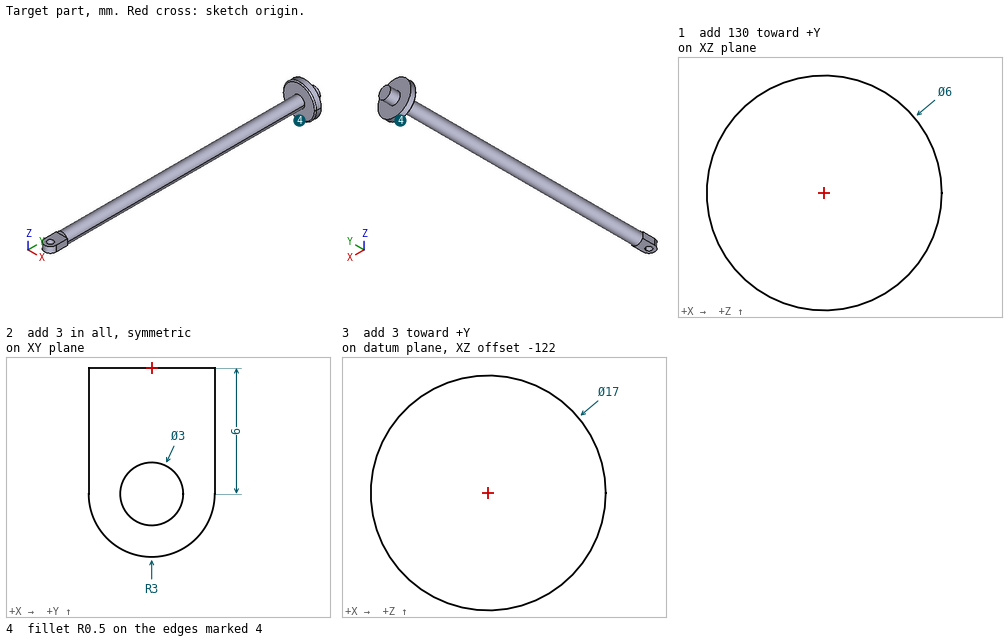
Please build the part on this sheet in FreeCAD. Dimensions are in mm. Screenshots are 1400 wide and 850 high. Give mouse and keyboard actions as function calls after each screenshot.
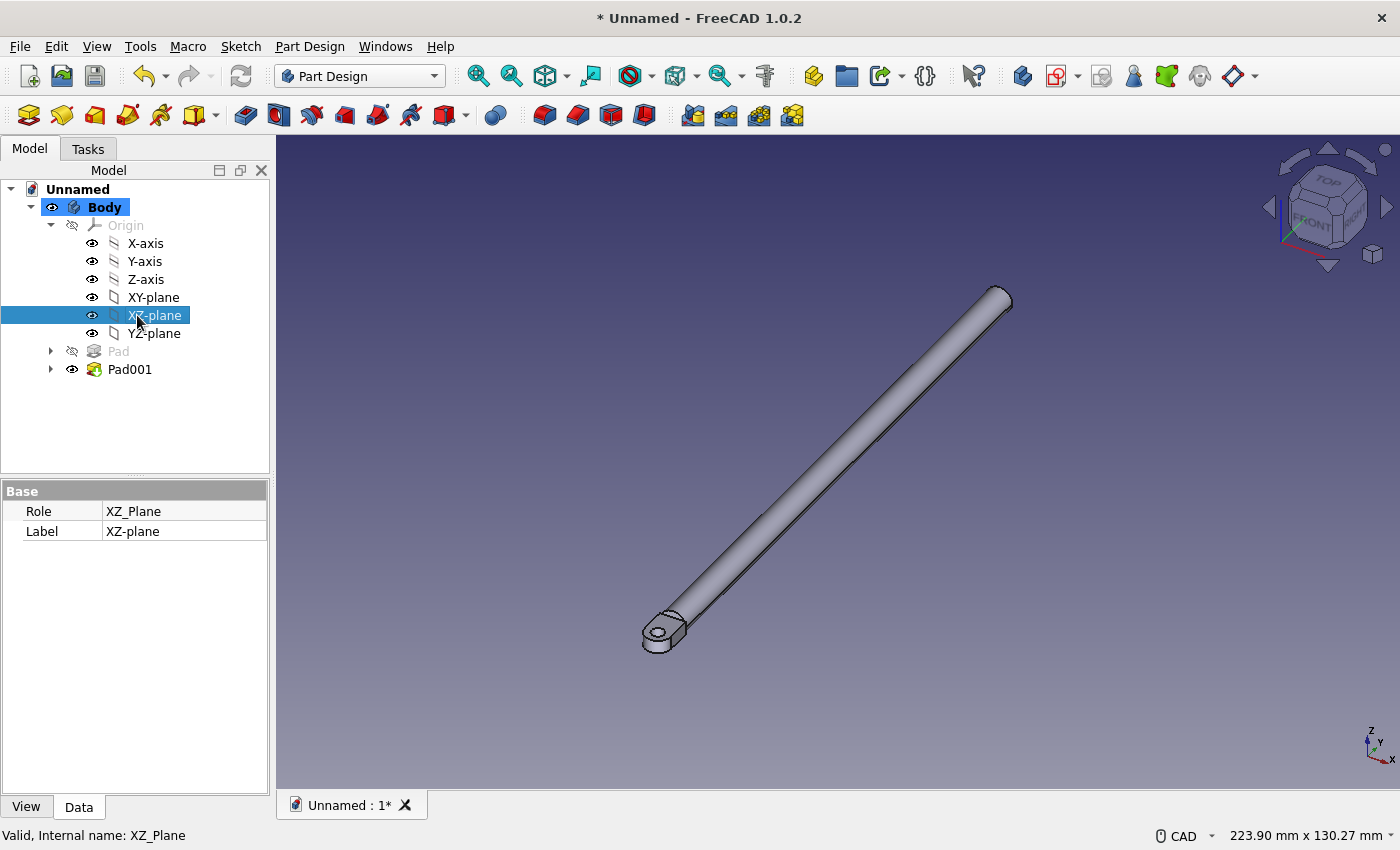
click(1232, 76)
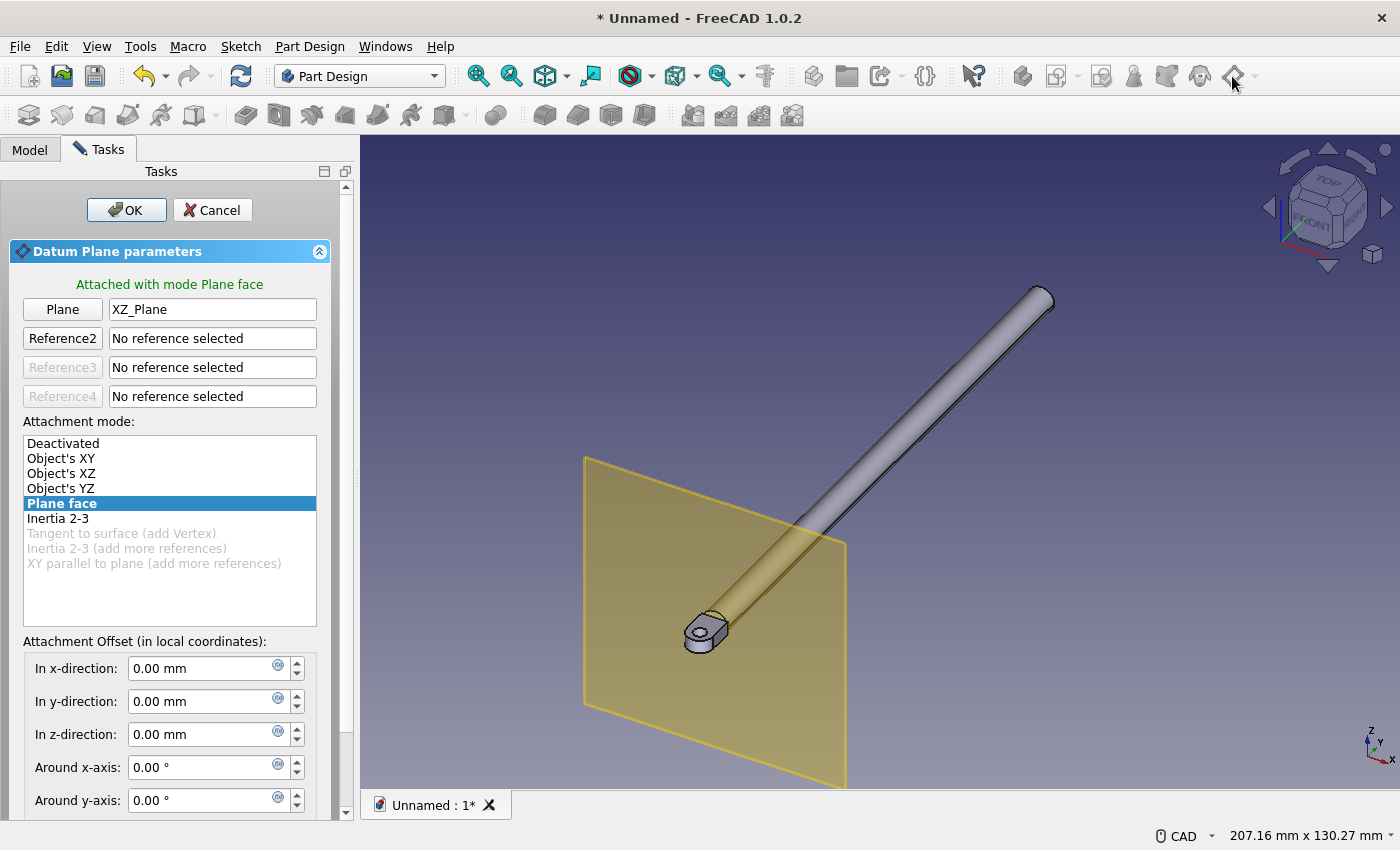
triple_click(210, 734)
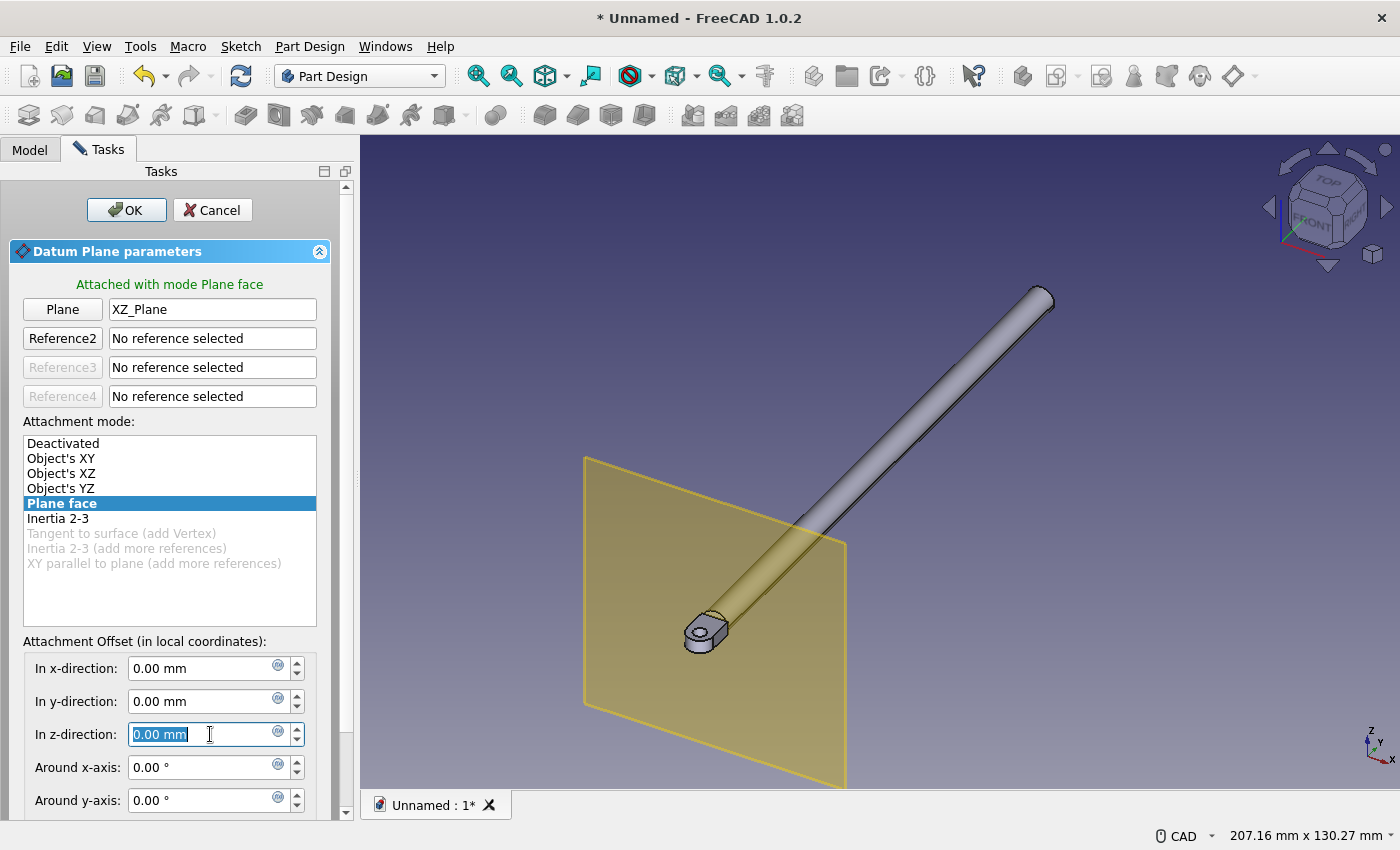
text(-122)
key(Tab)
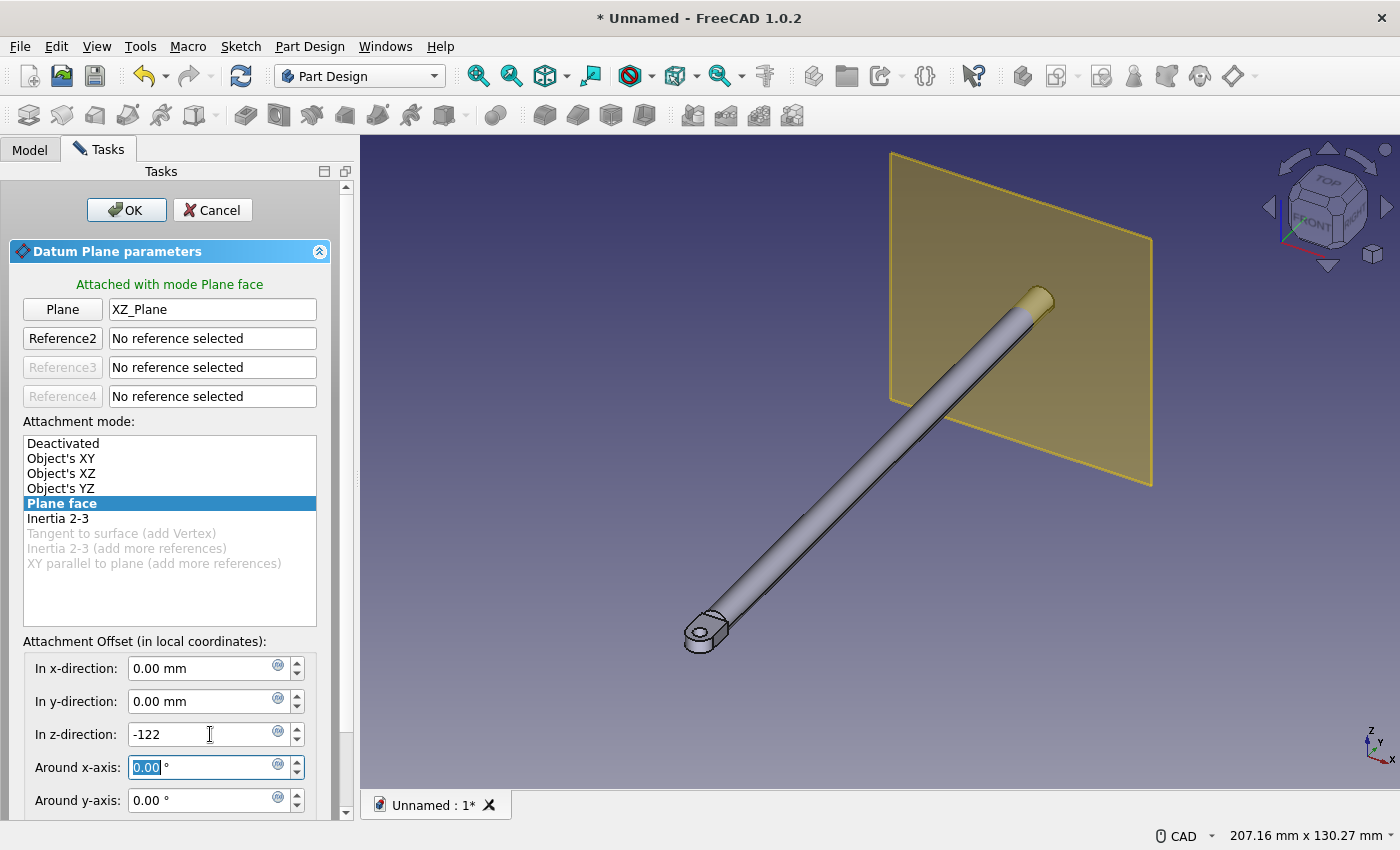
click(127, 210)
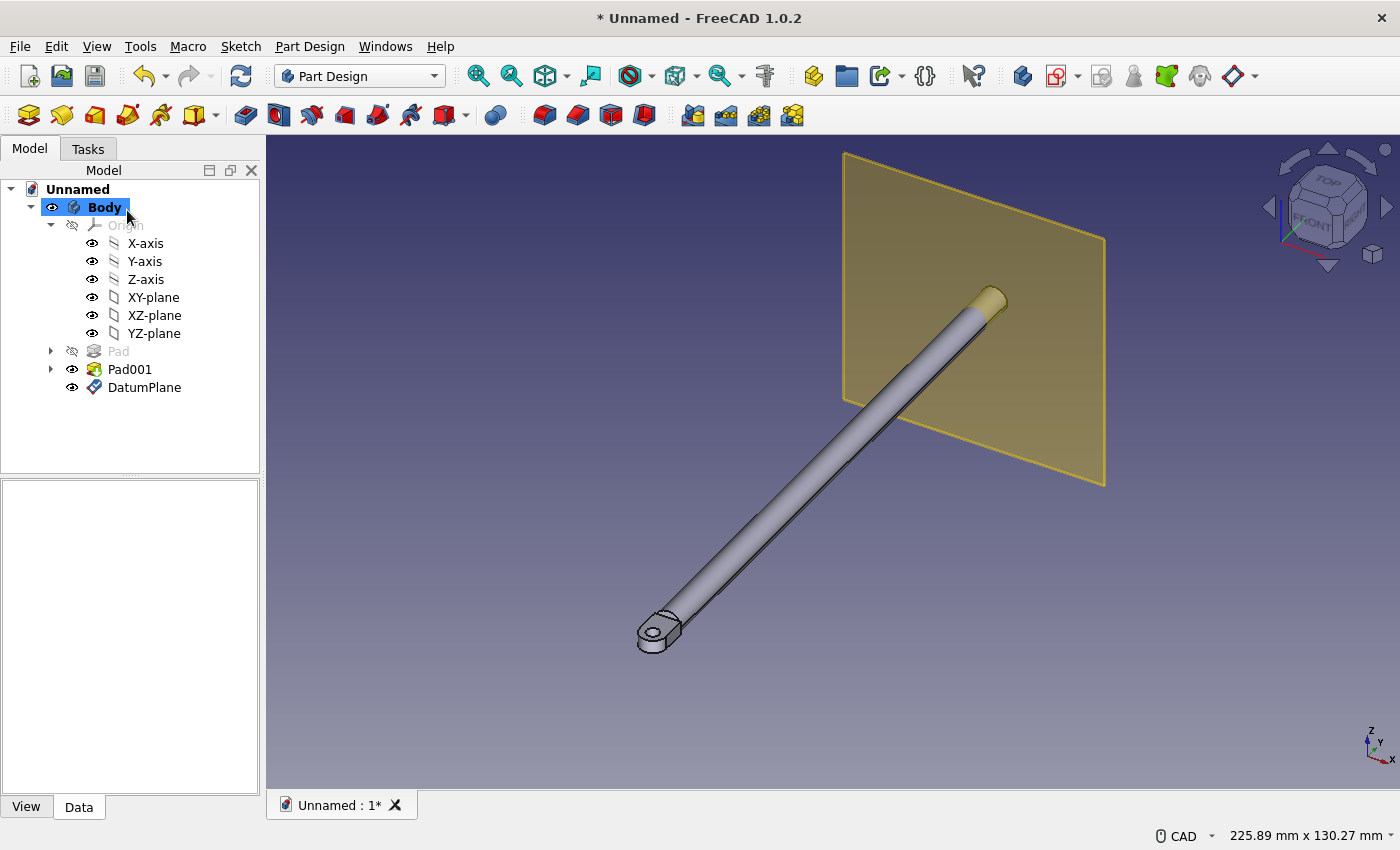
click(117, 387)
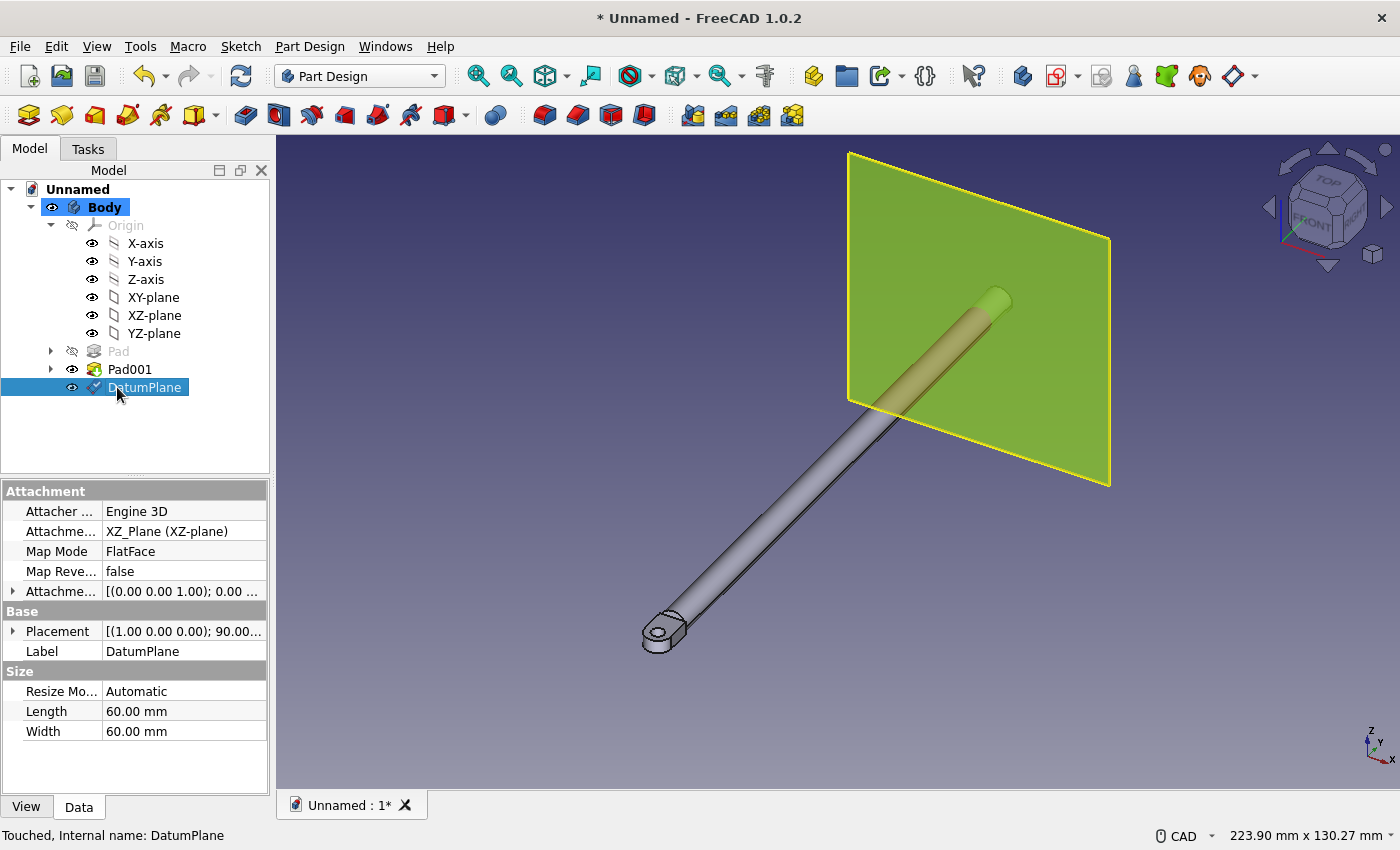
click(1056, 76)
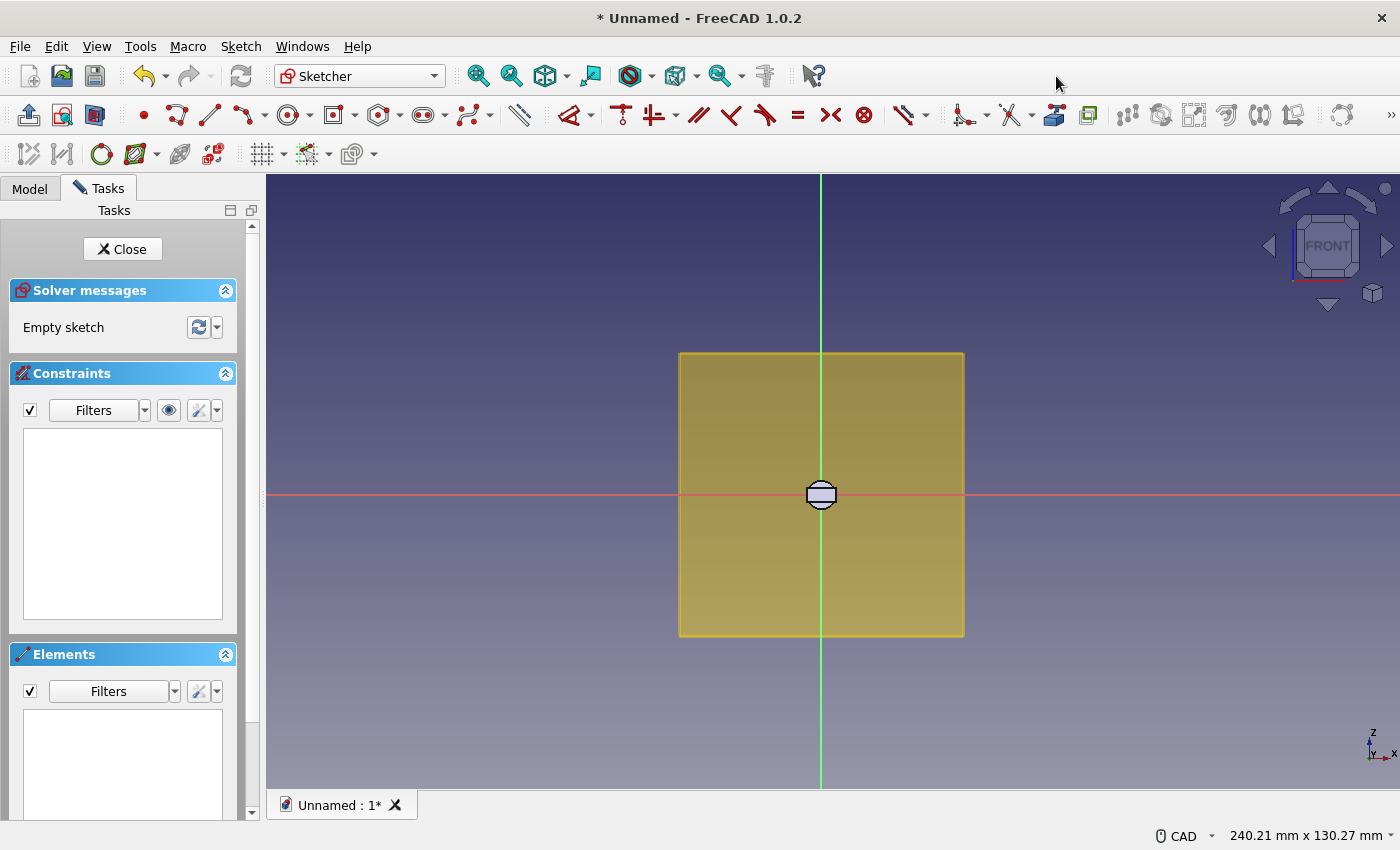
key(q)
key(s)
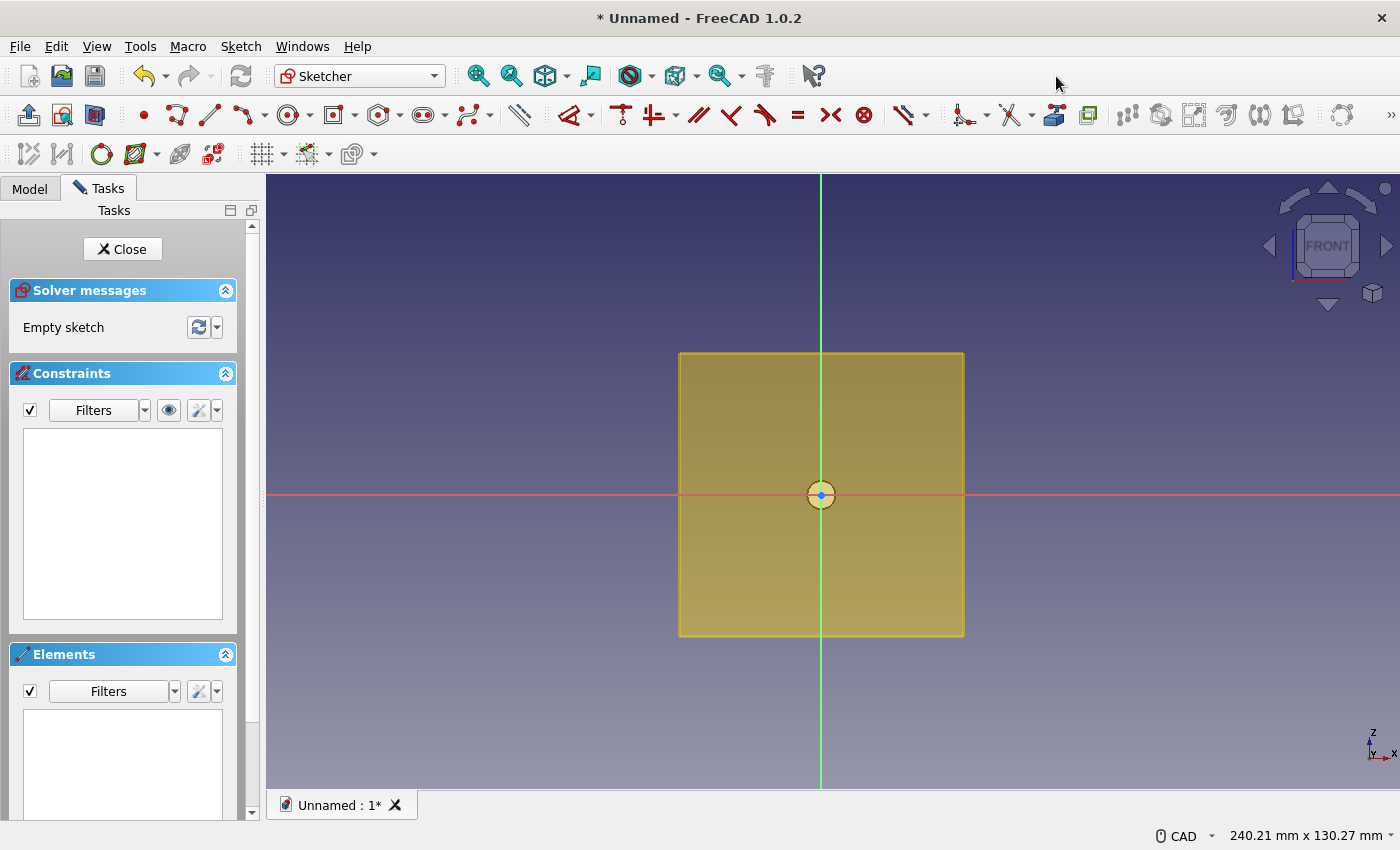
scroll(836, 498, up, 8)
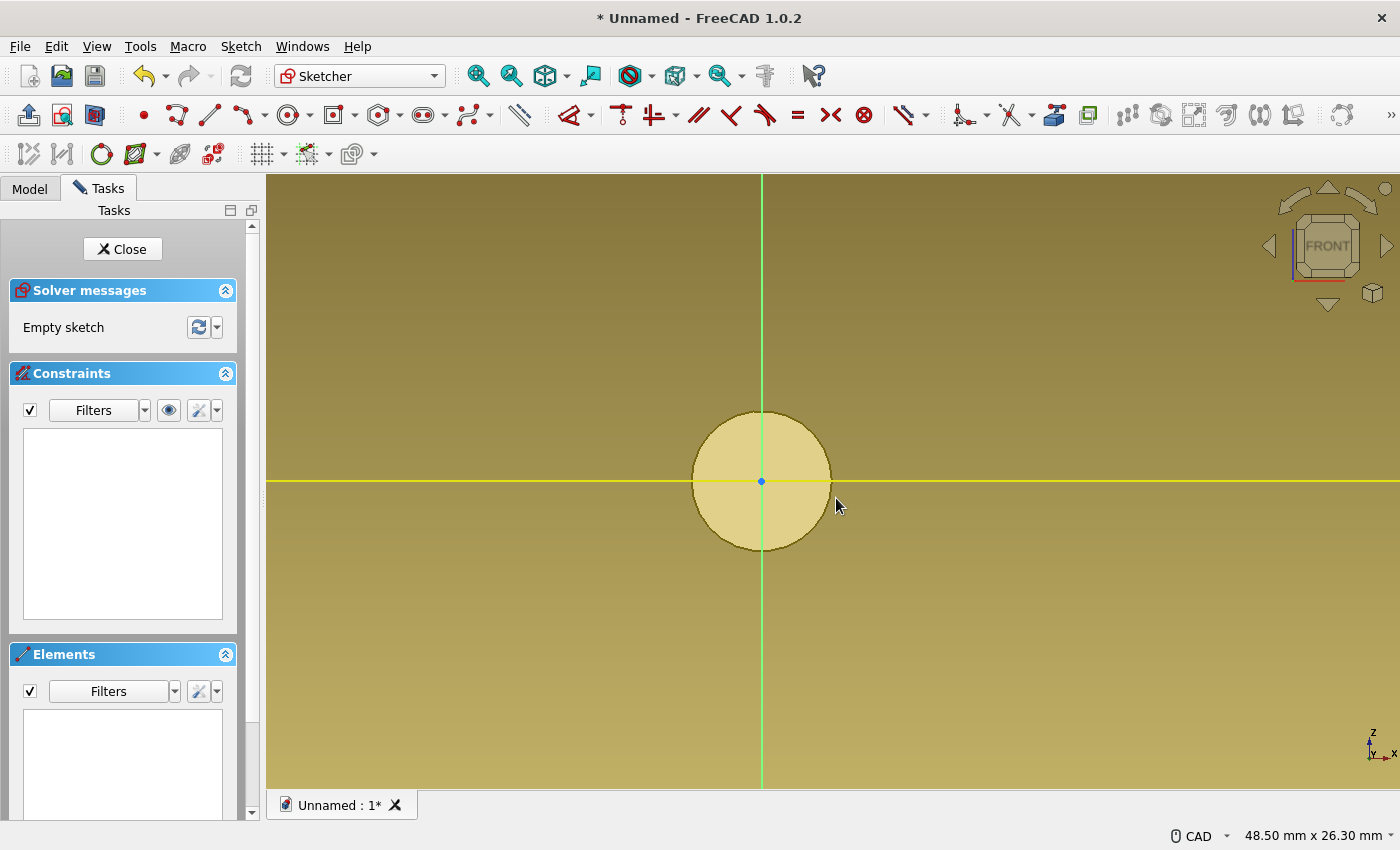
key(g)
key(c)